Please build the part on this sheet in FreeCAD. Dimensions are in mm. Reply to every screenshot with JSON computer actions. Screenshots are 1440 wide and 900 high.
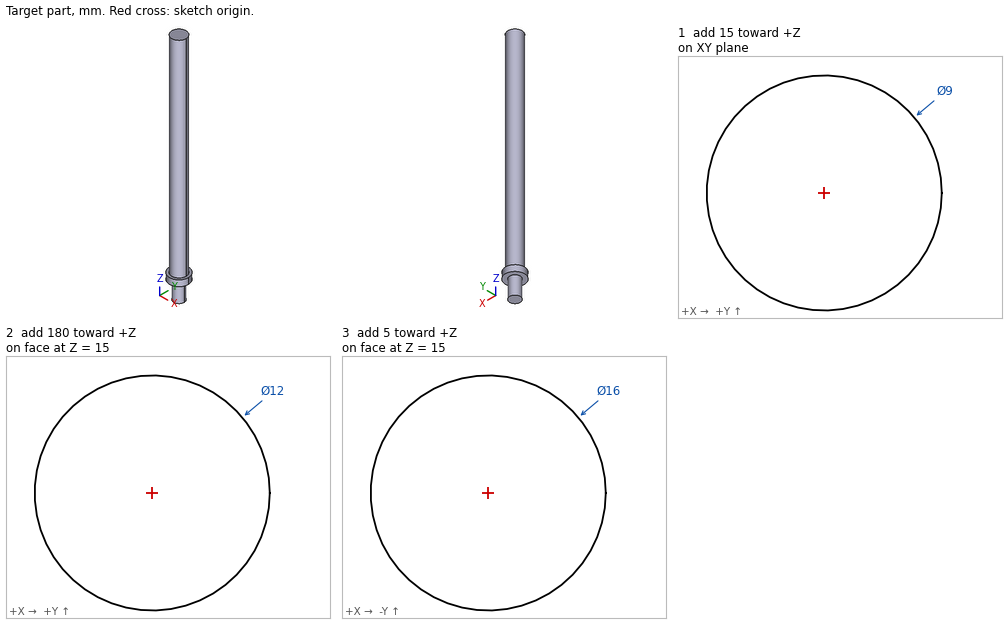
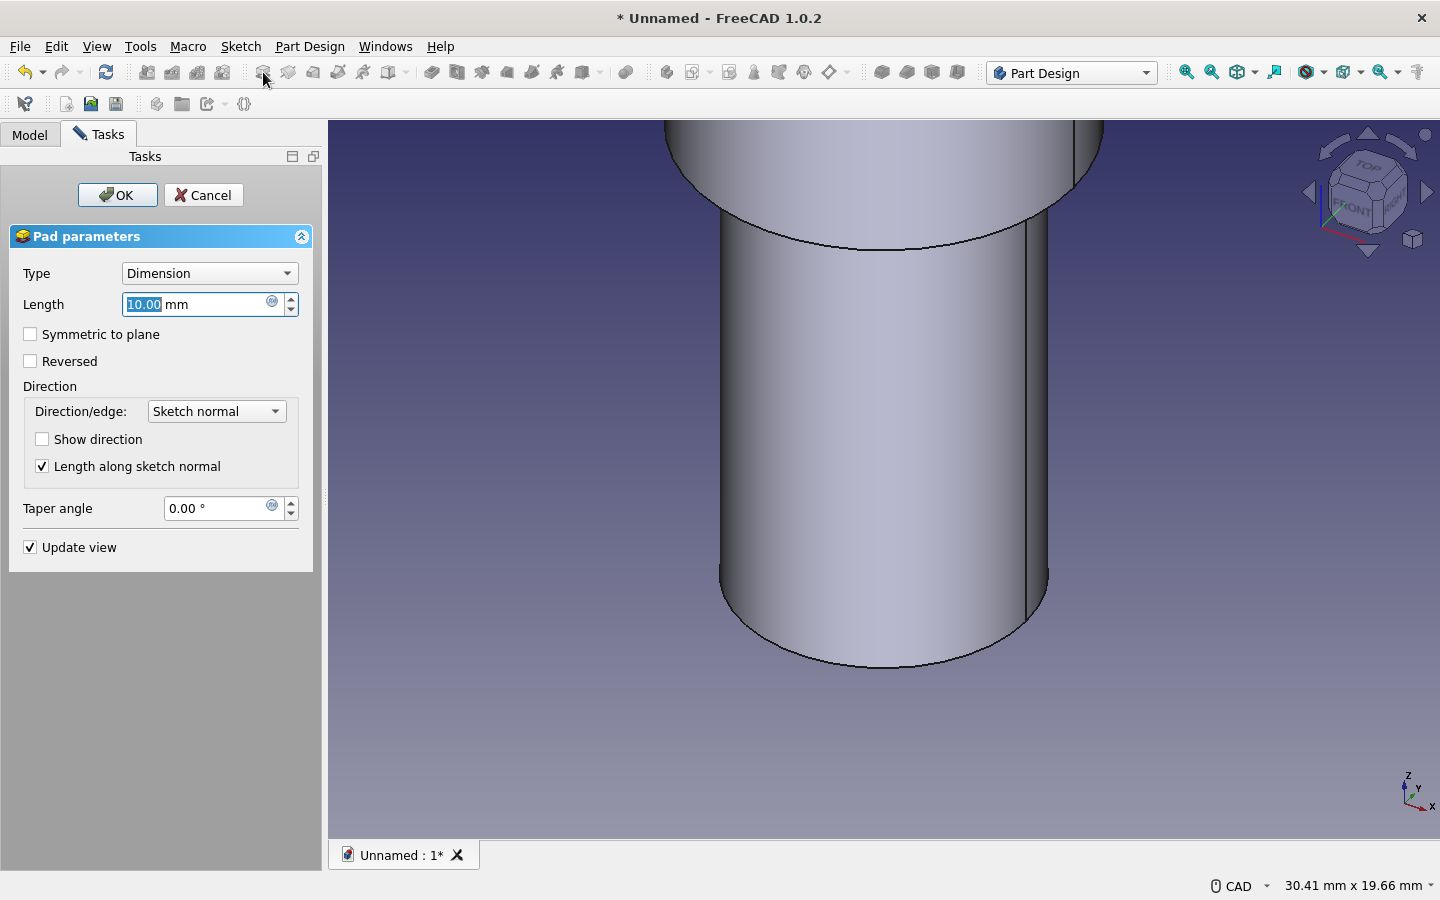
{"action": "type", "text": "180"}
{"action": "key", "text": "Tab"}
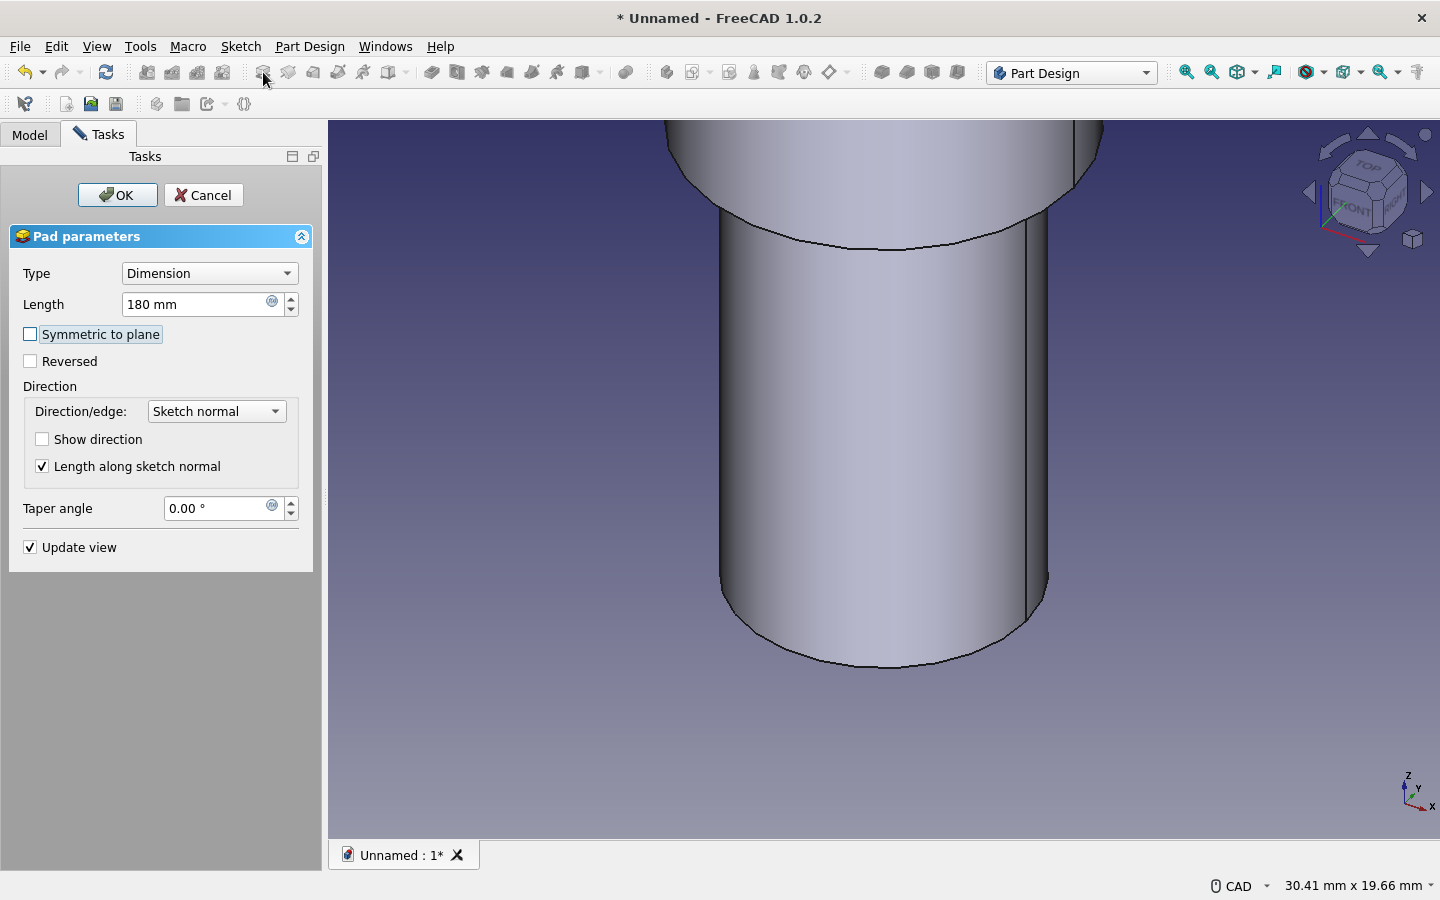
{"action": "left_click", "coordinate": [118, 195]}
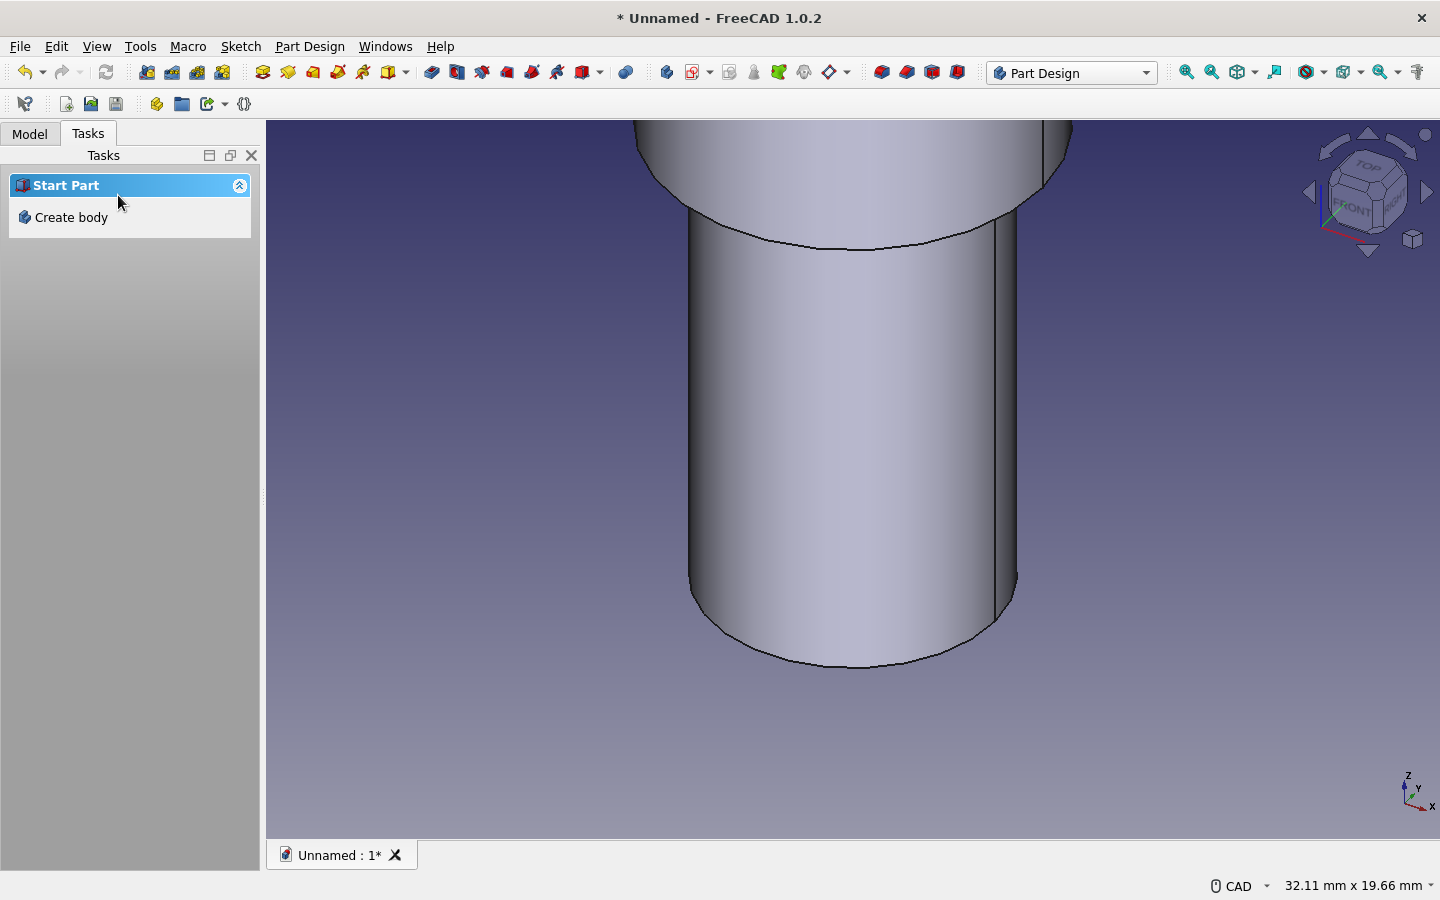
{"action": "key", "text": "v f"}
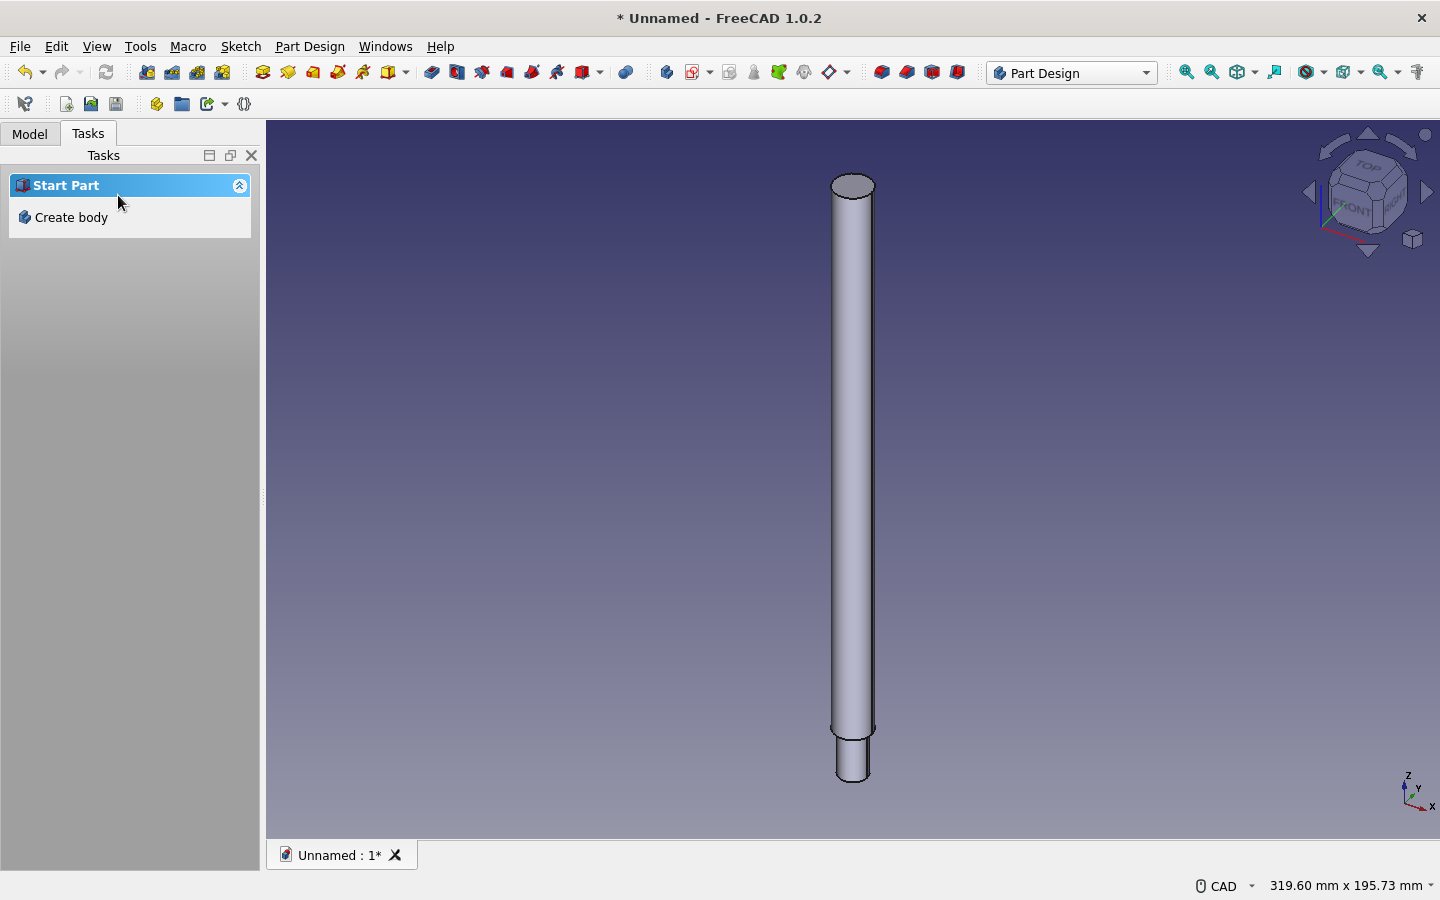
{"action": "key", "text": "5"}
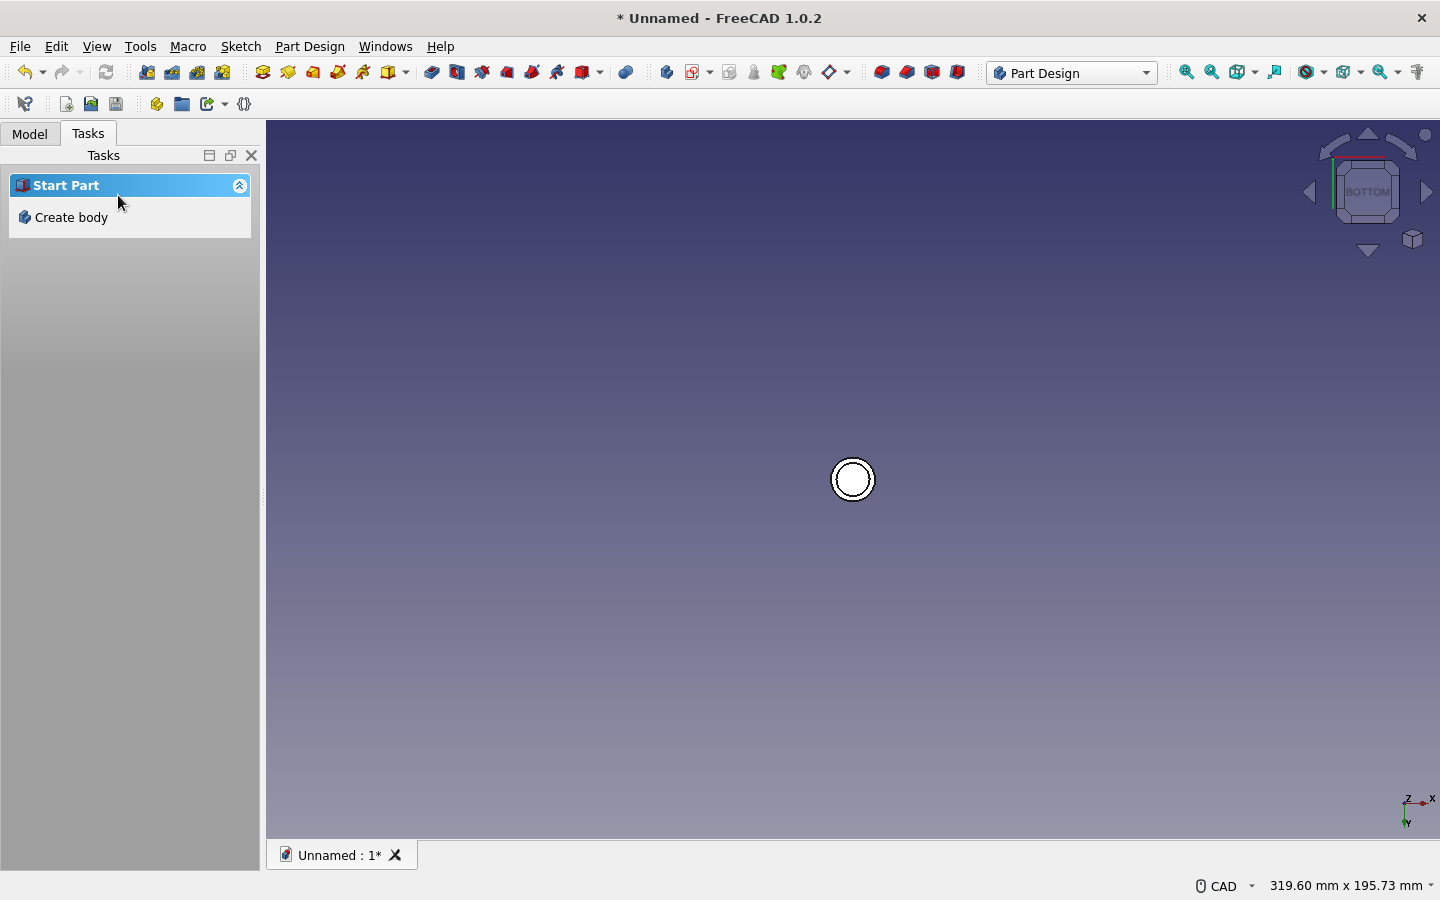
{"action": "key", "text": "v f"}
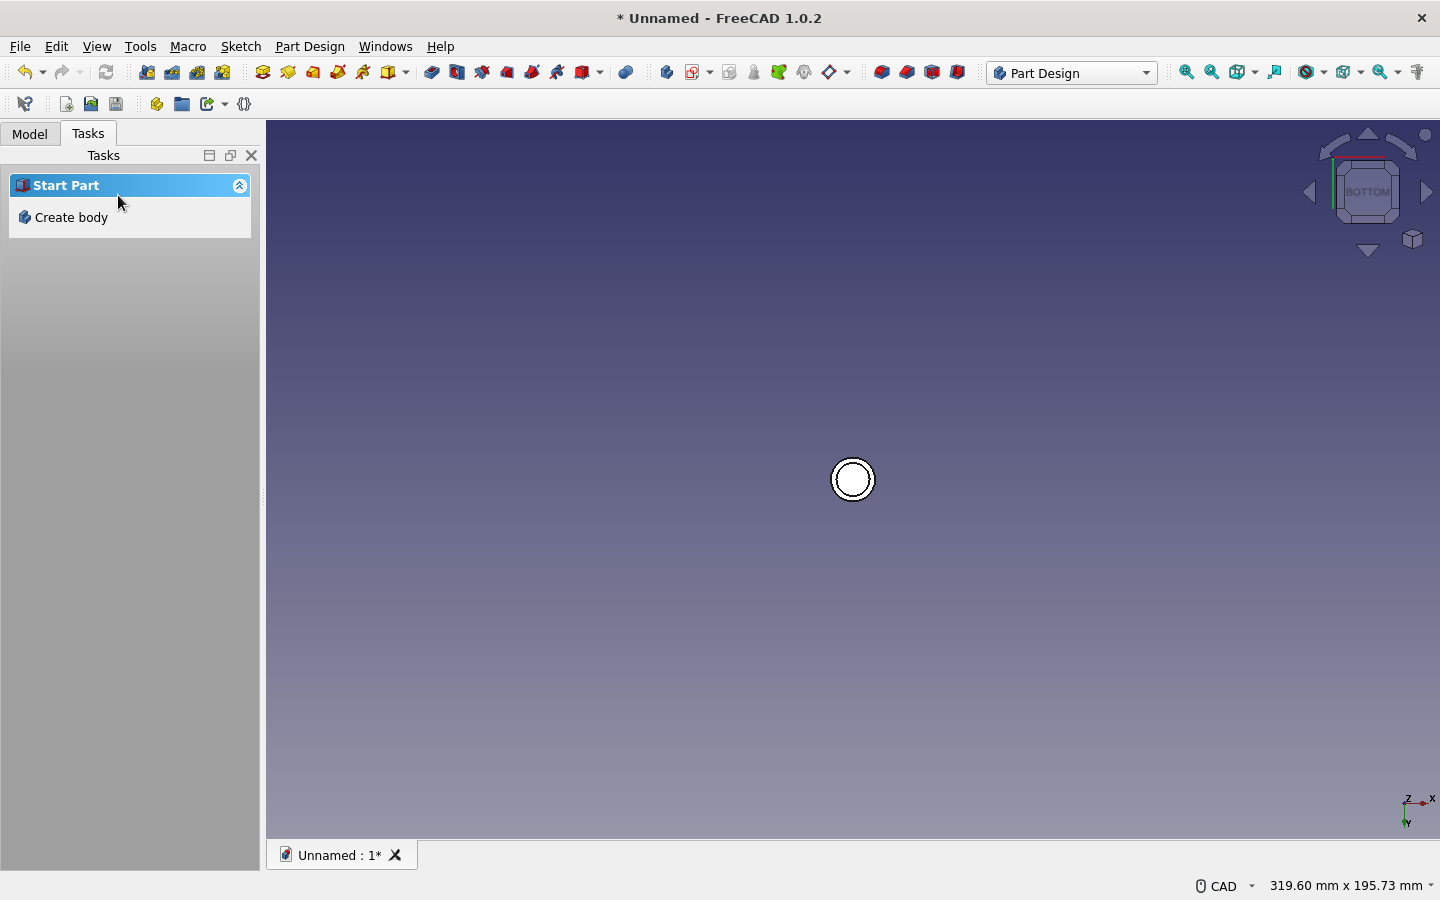
{"action": "scroll", "coordinate": [853, 460], "scroll_direction": "up", "scroll_amount": 9}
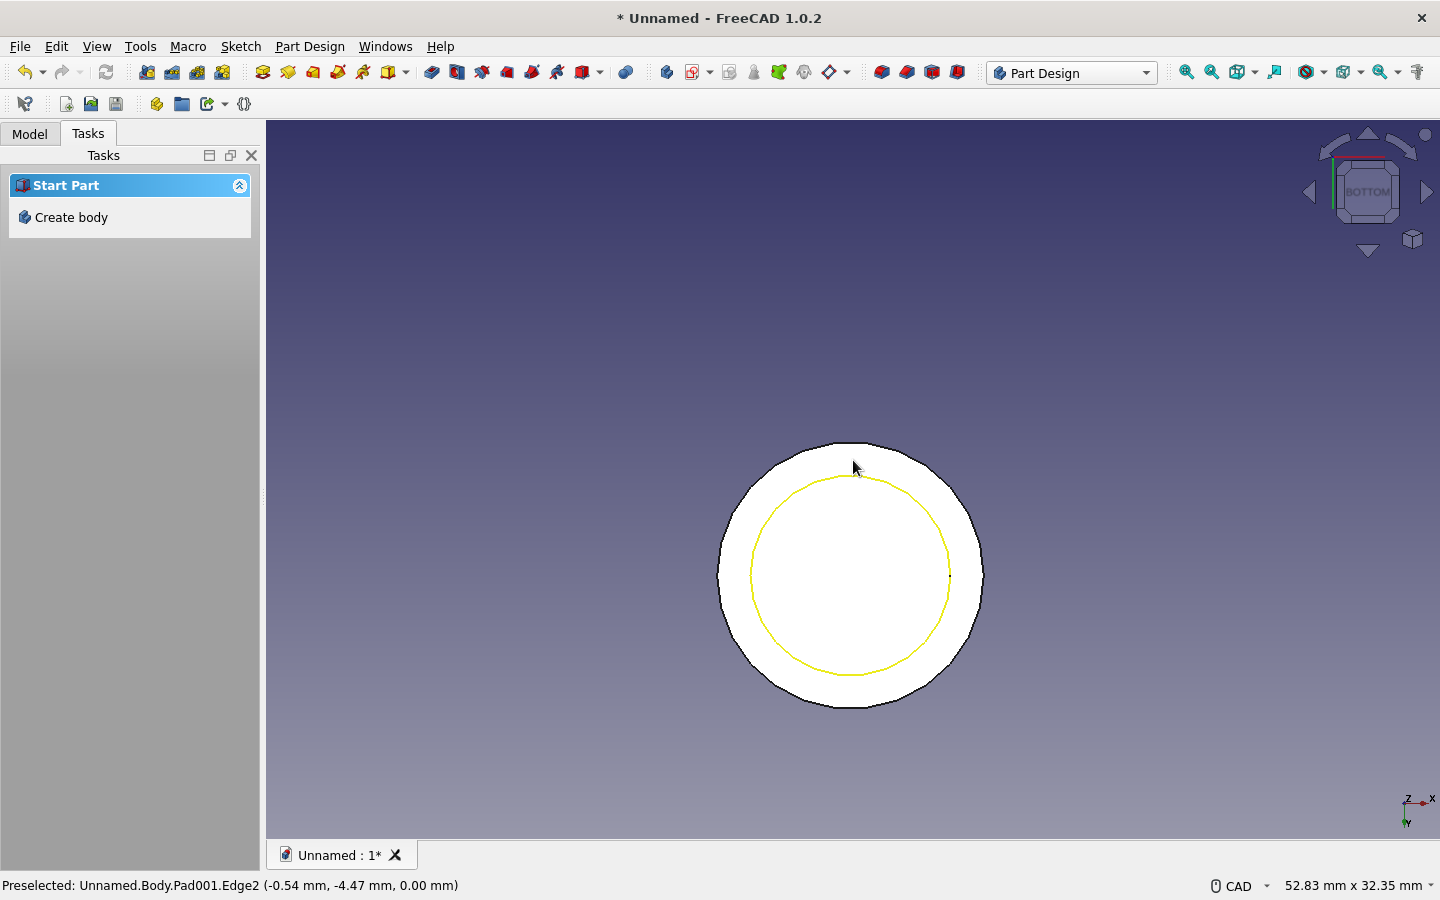
{"action": "left_click", "coordinate": [850, 460]}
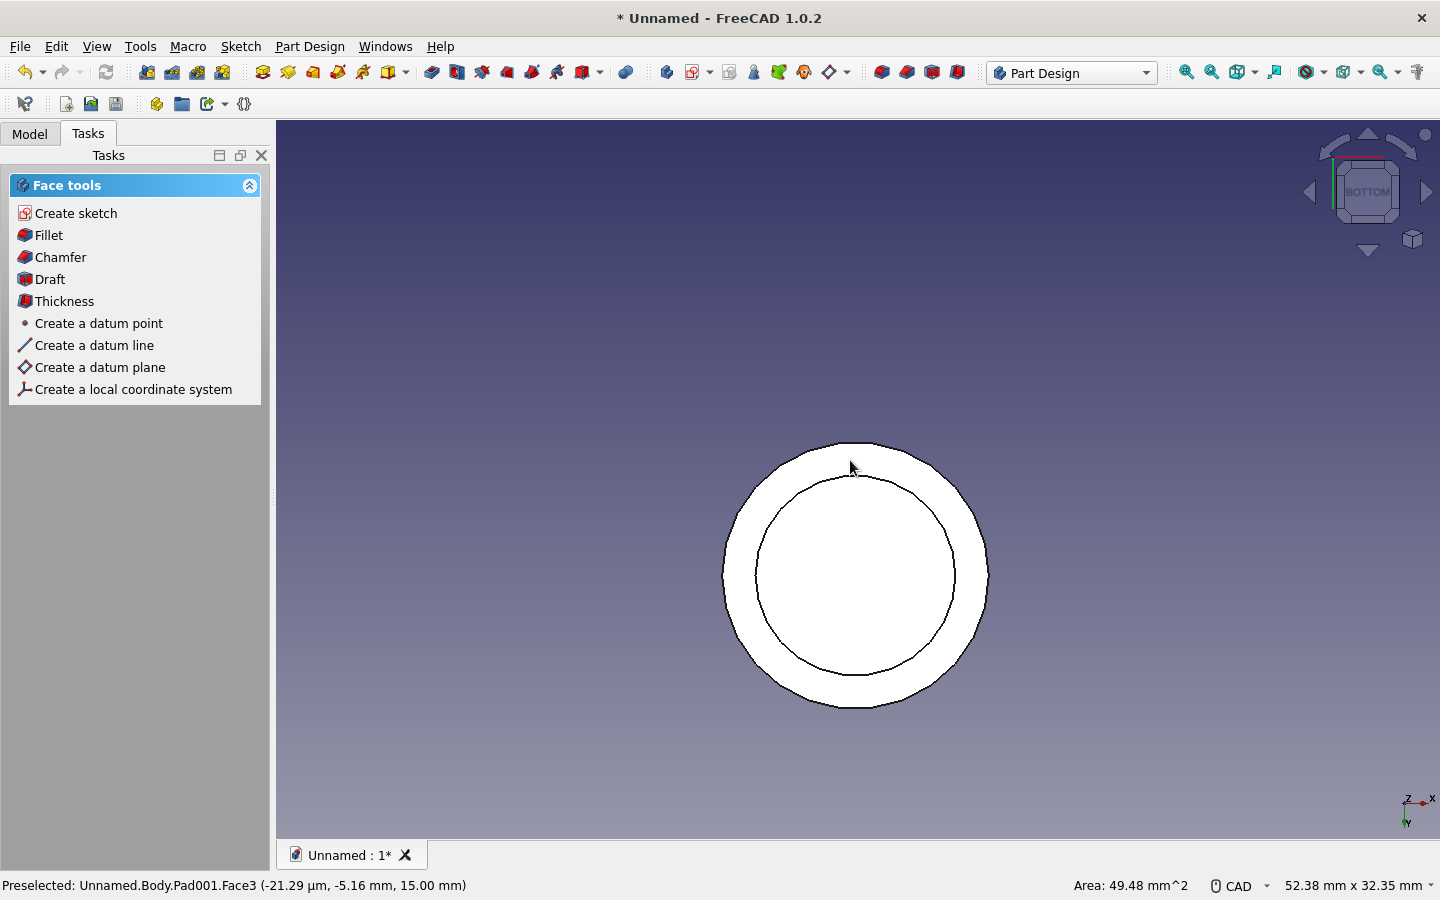
{"action": "left_click", "coordinate": [692, 72]}